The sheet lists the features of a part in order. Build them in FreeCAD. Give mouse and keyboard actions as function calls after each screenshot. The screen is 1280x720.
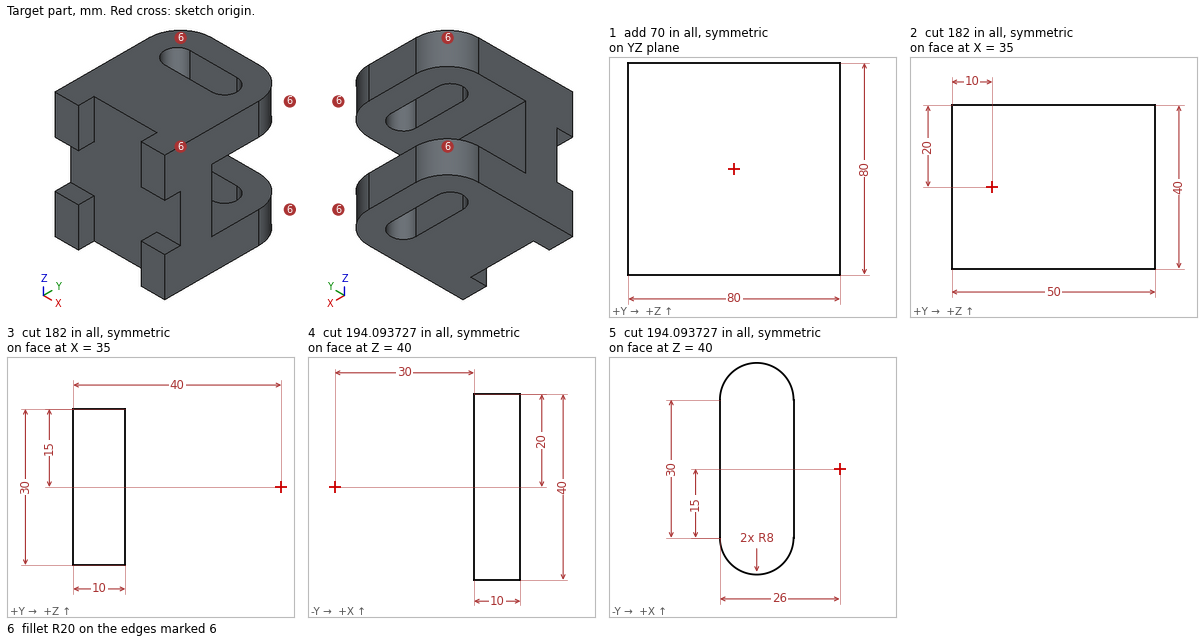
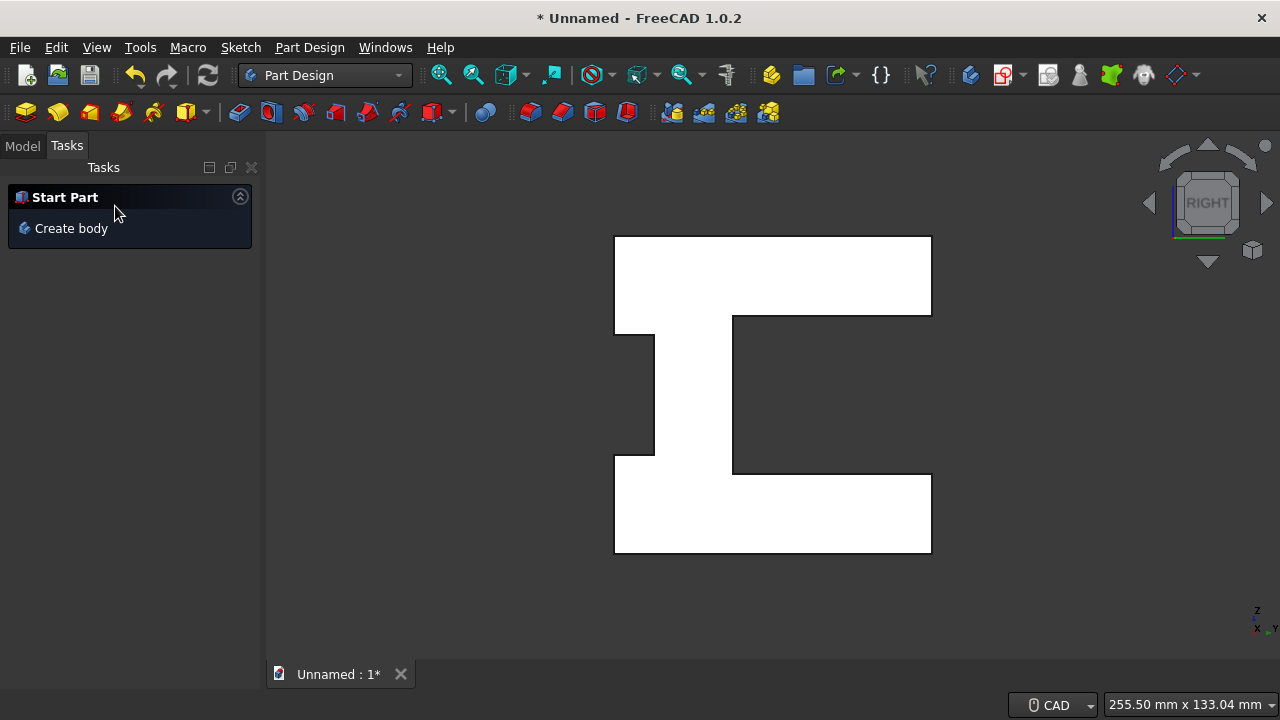
click(932, 275)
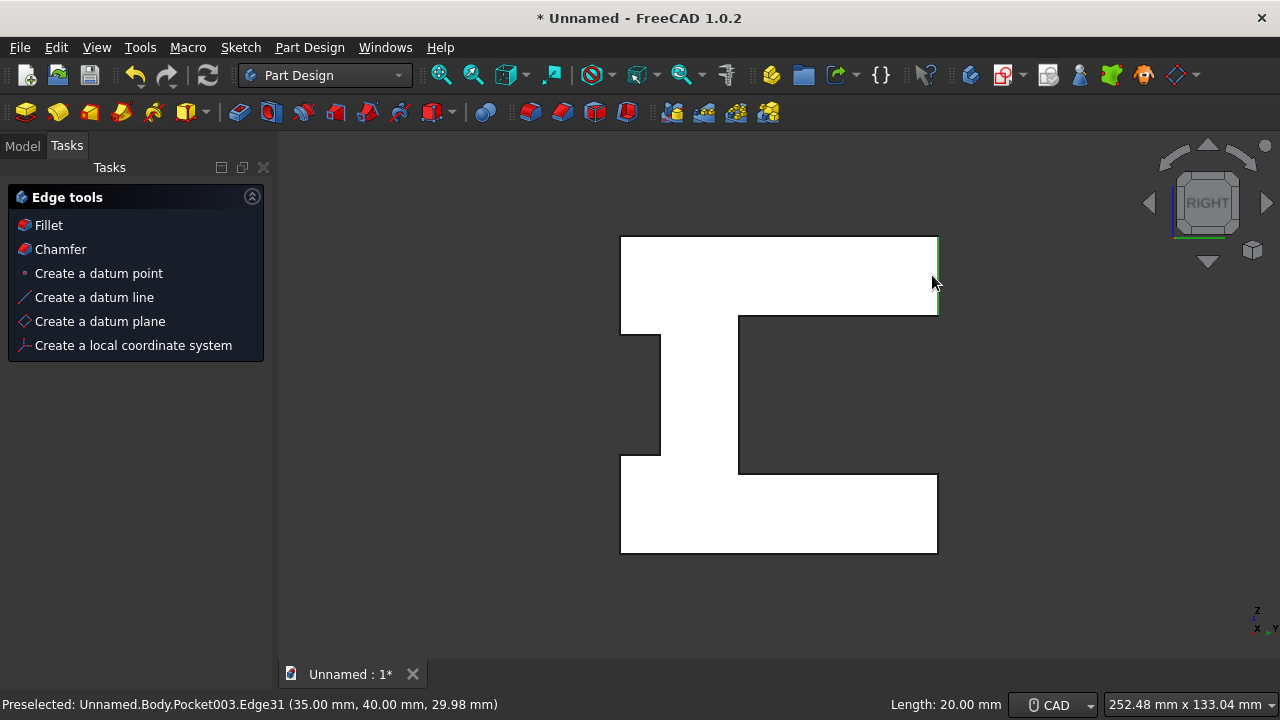
click(938, 513, ctrl)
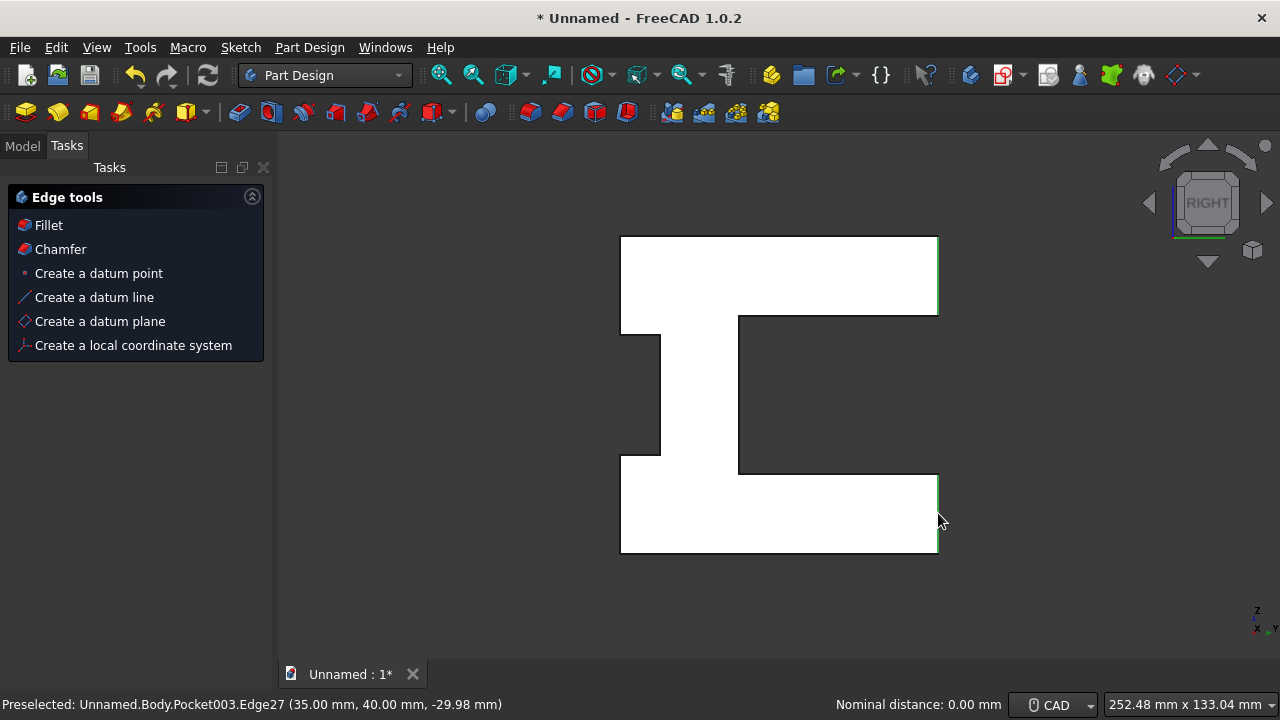
key(5)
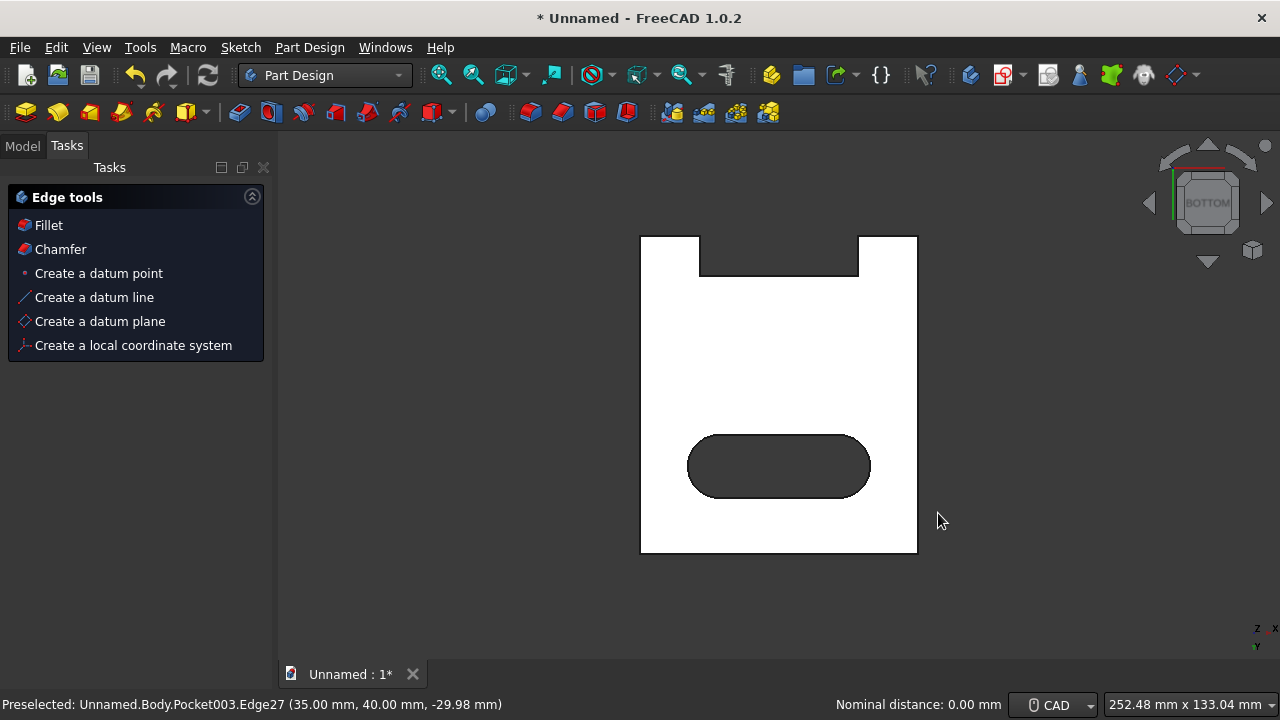
key(4)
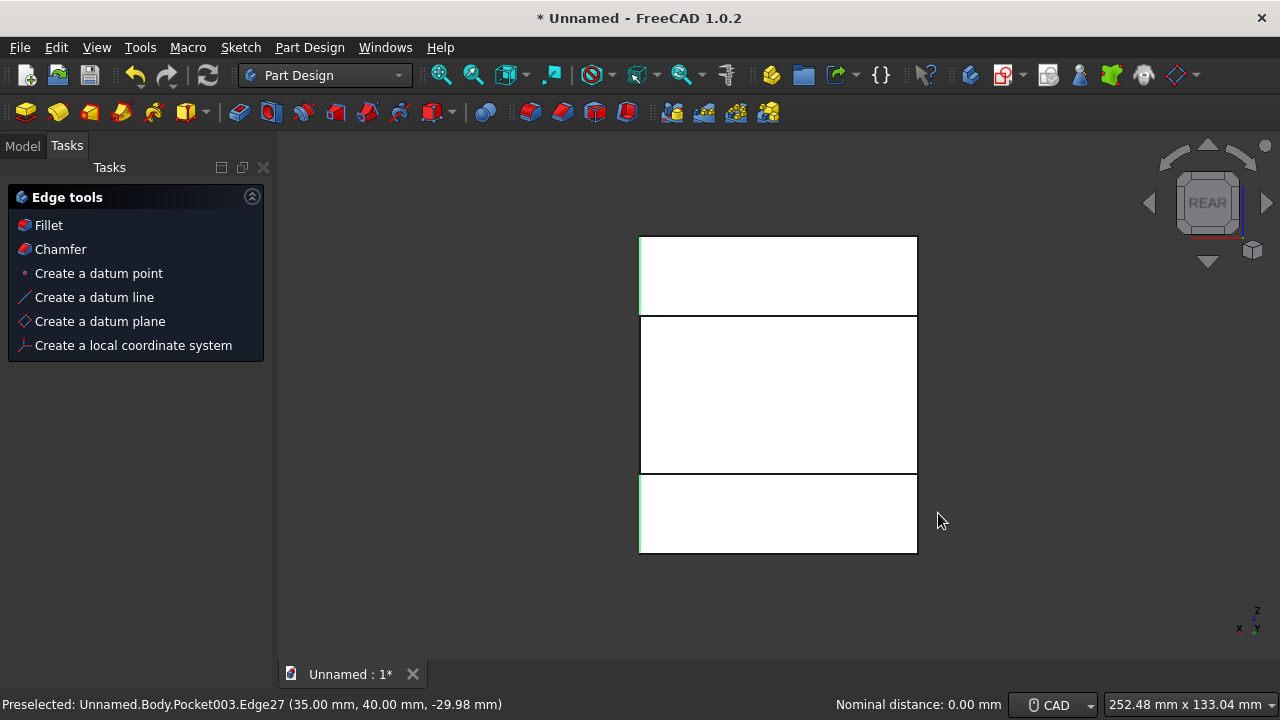
click(918, 275, ctrl)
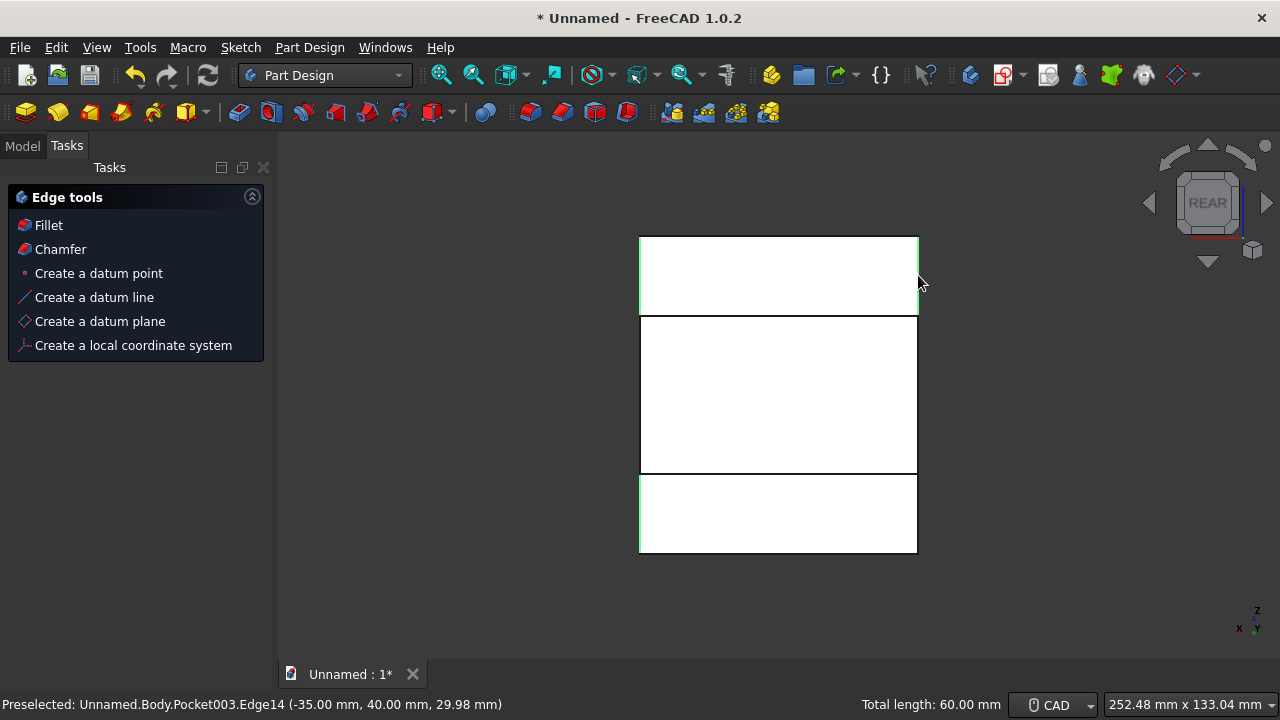
click(918, 513, ctrl)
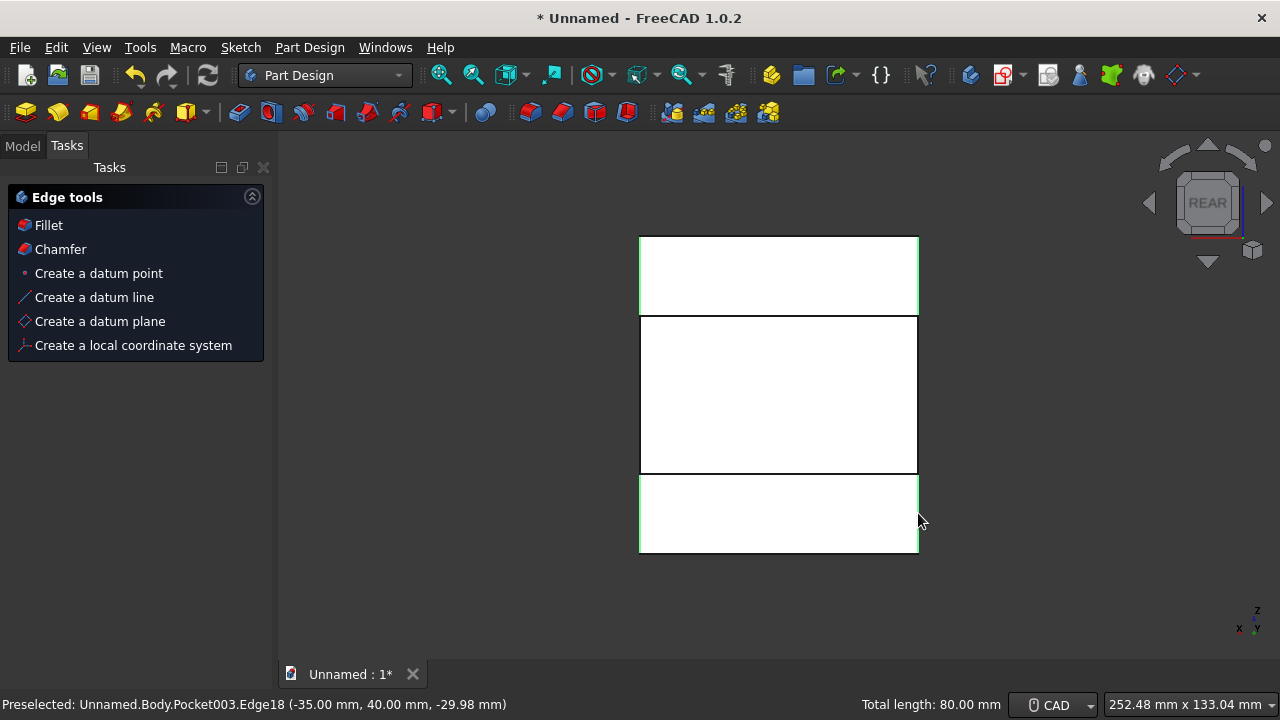
click(532, 112)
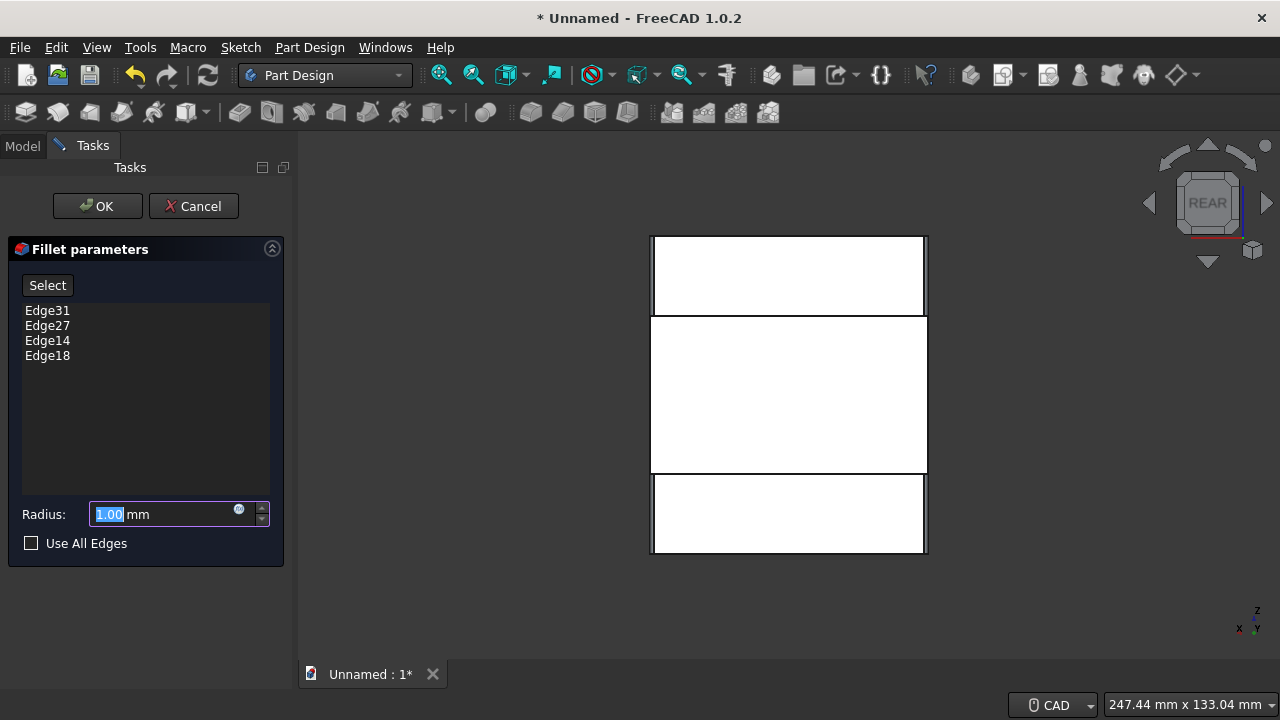
text(20)
key(Tab)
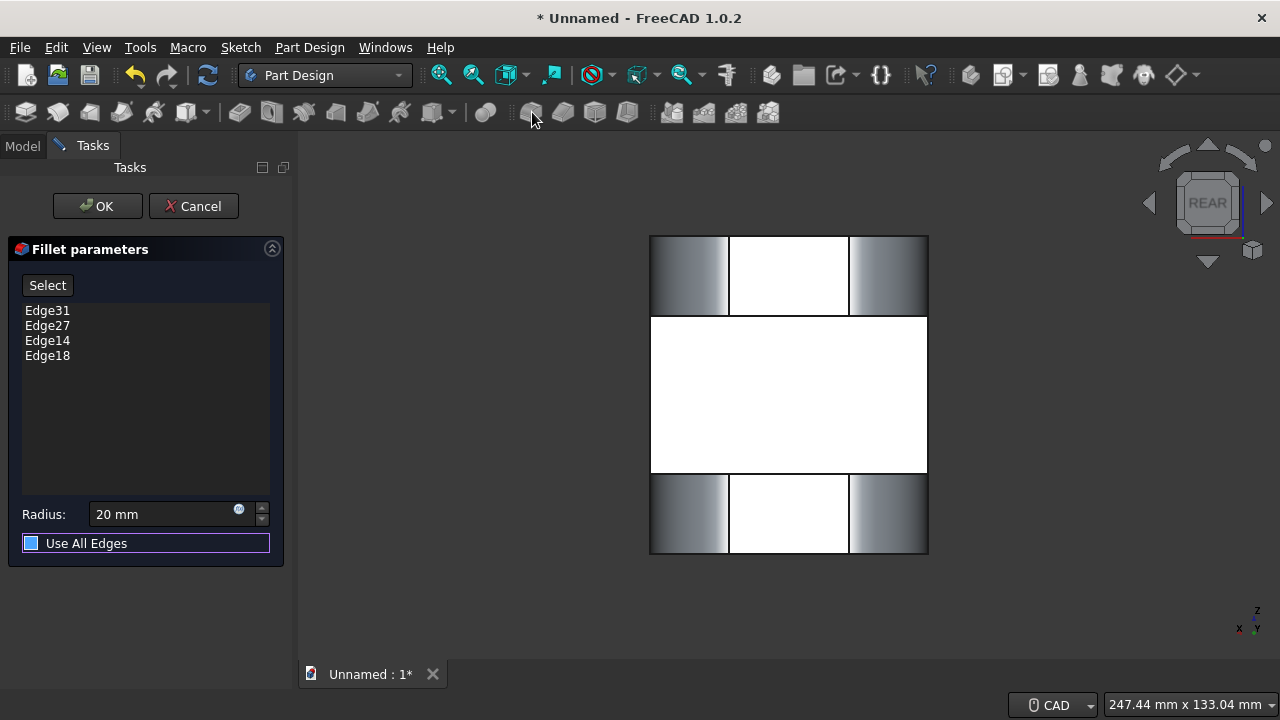
click(98, 206)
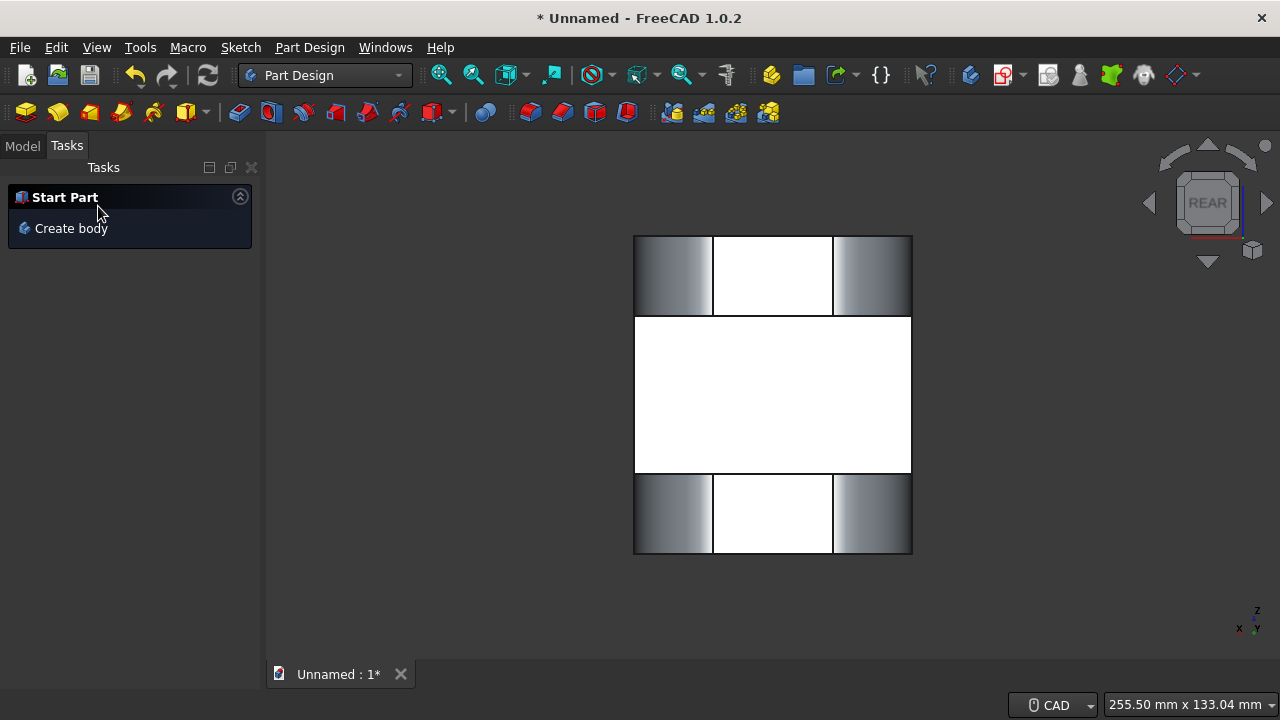
key(0)